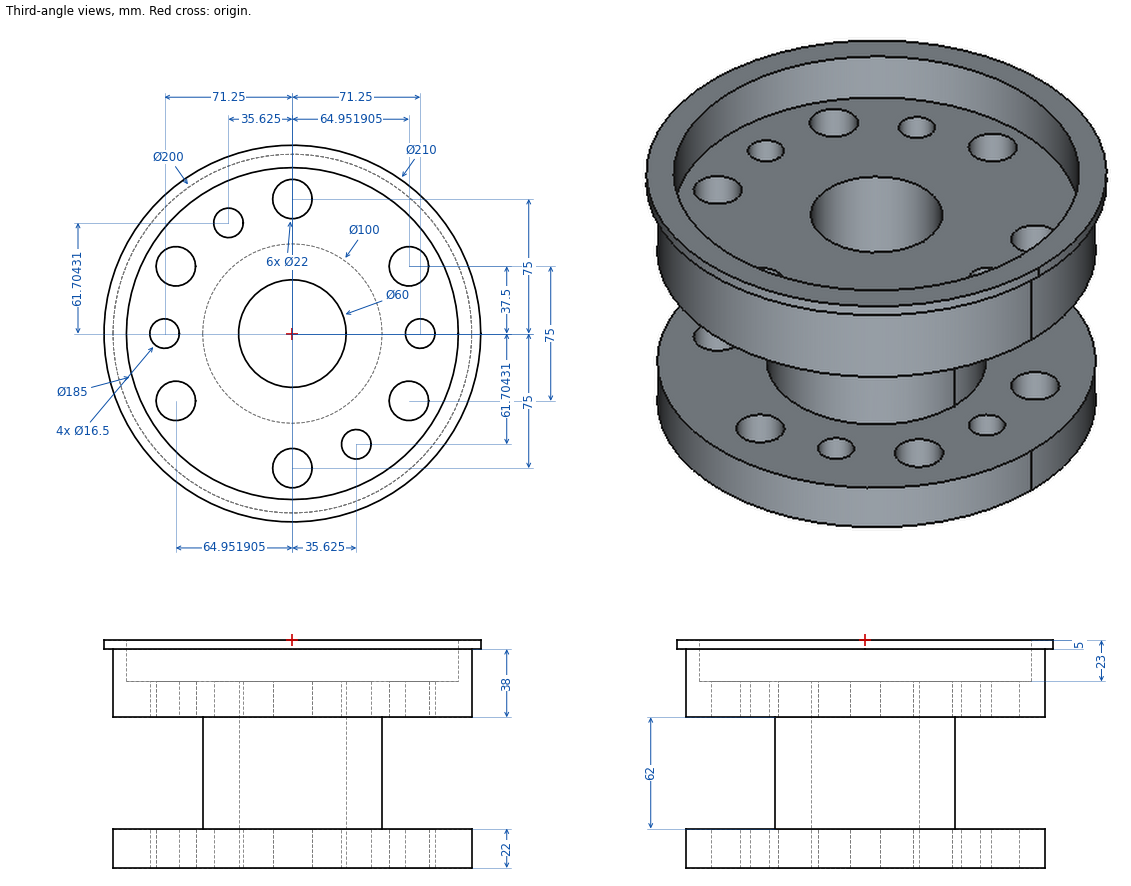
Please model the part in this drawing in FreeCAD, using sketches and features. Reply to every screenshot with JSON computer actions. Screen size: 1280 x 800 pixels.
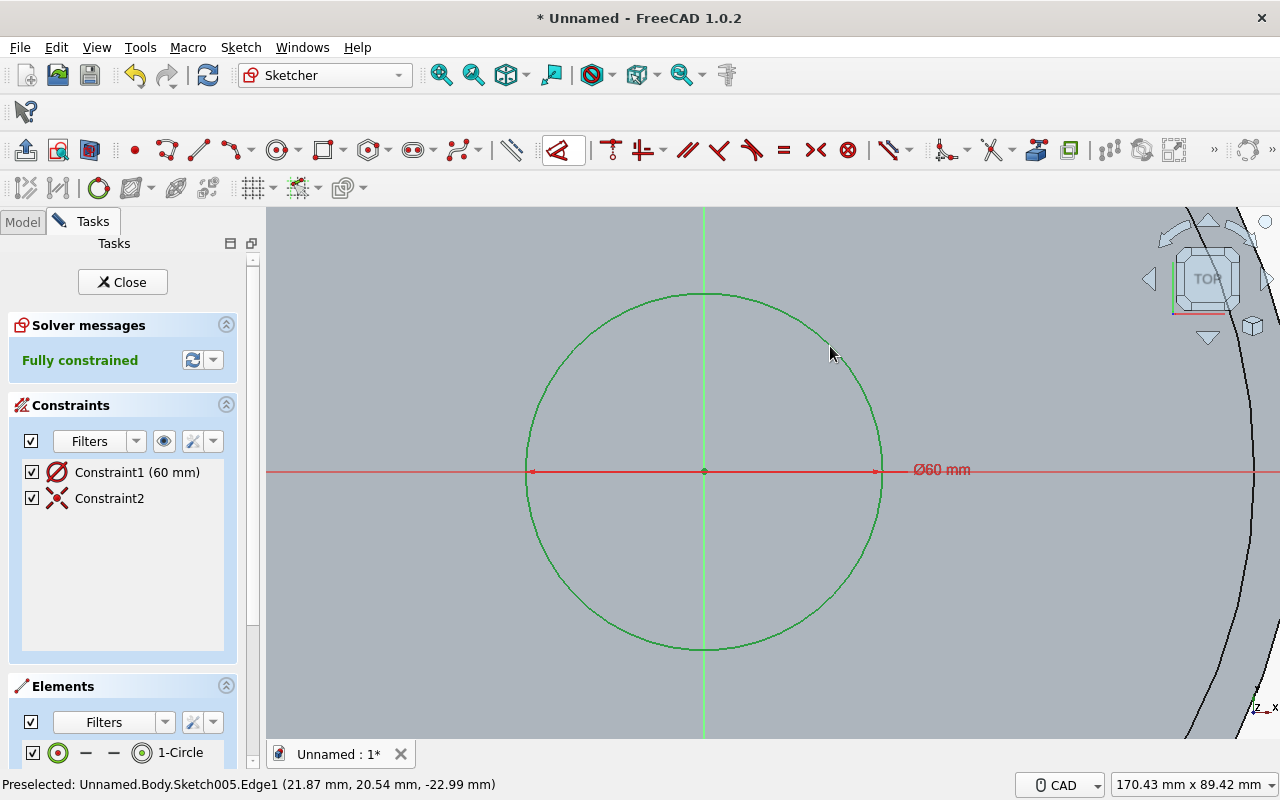
{"action": "left_click", "coordinate": [123, 282]}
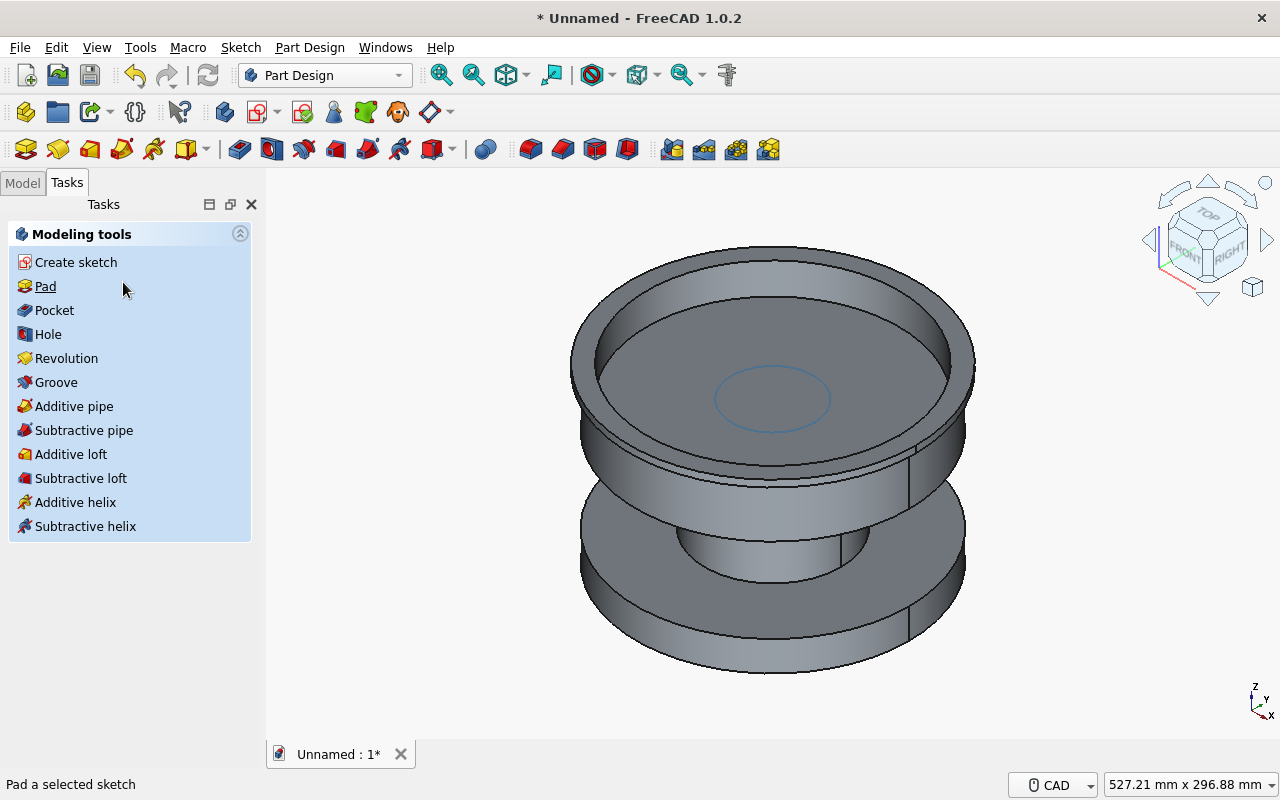
{"action": "left_click", "coordinate": [240, 150]}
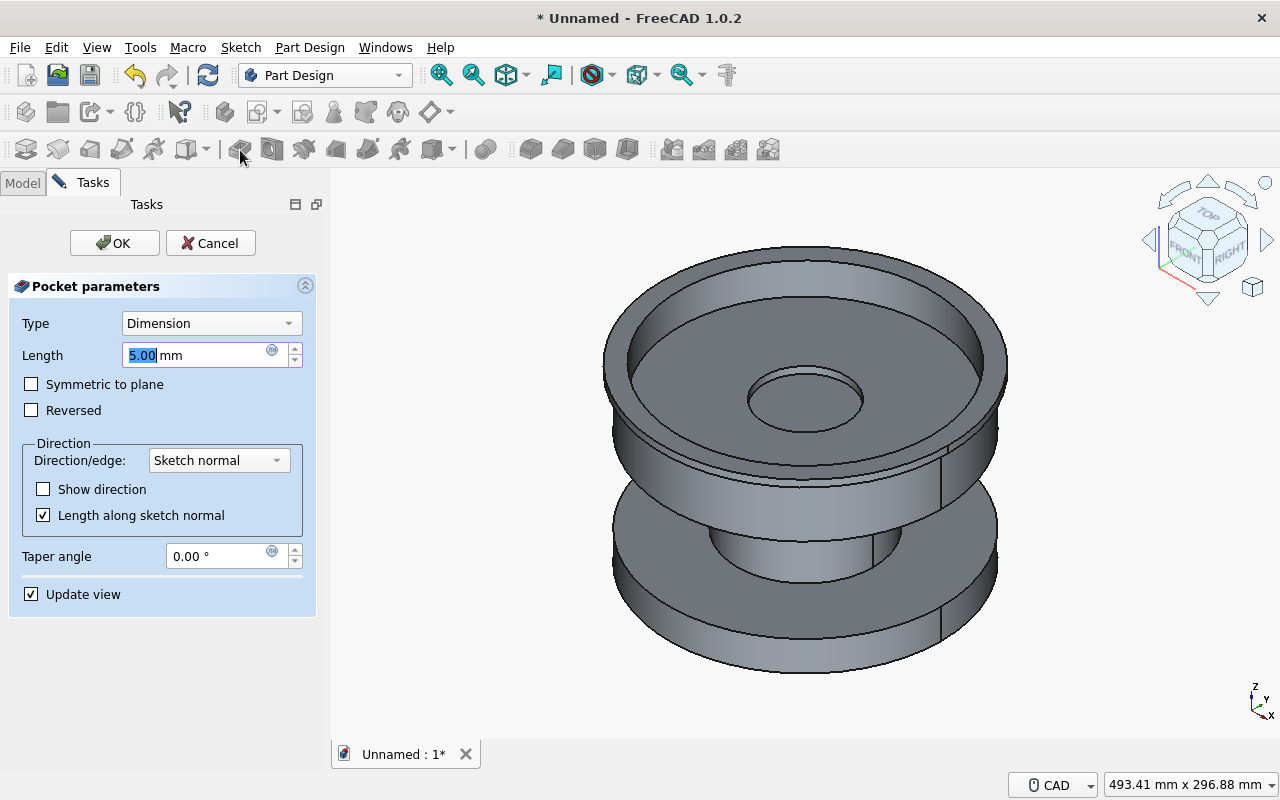
{"action": "left_click", "coordinate": [212, 324]}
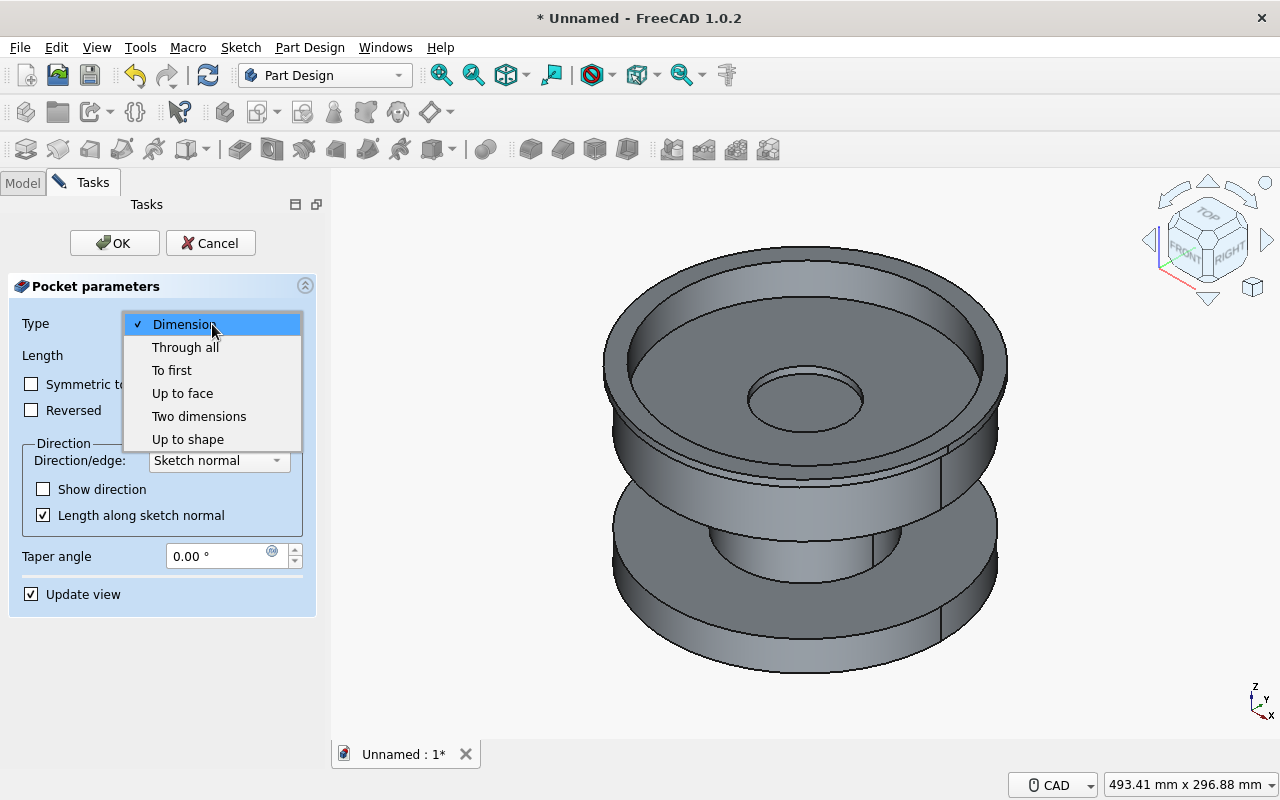
{"action": "left_click", "coordinate": [212, 348]}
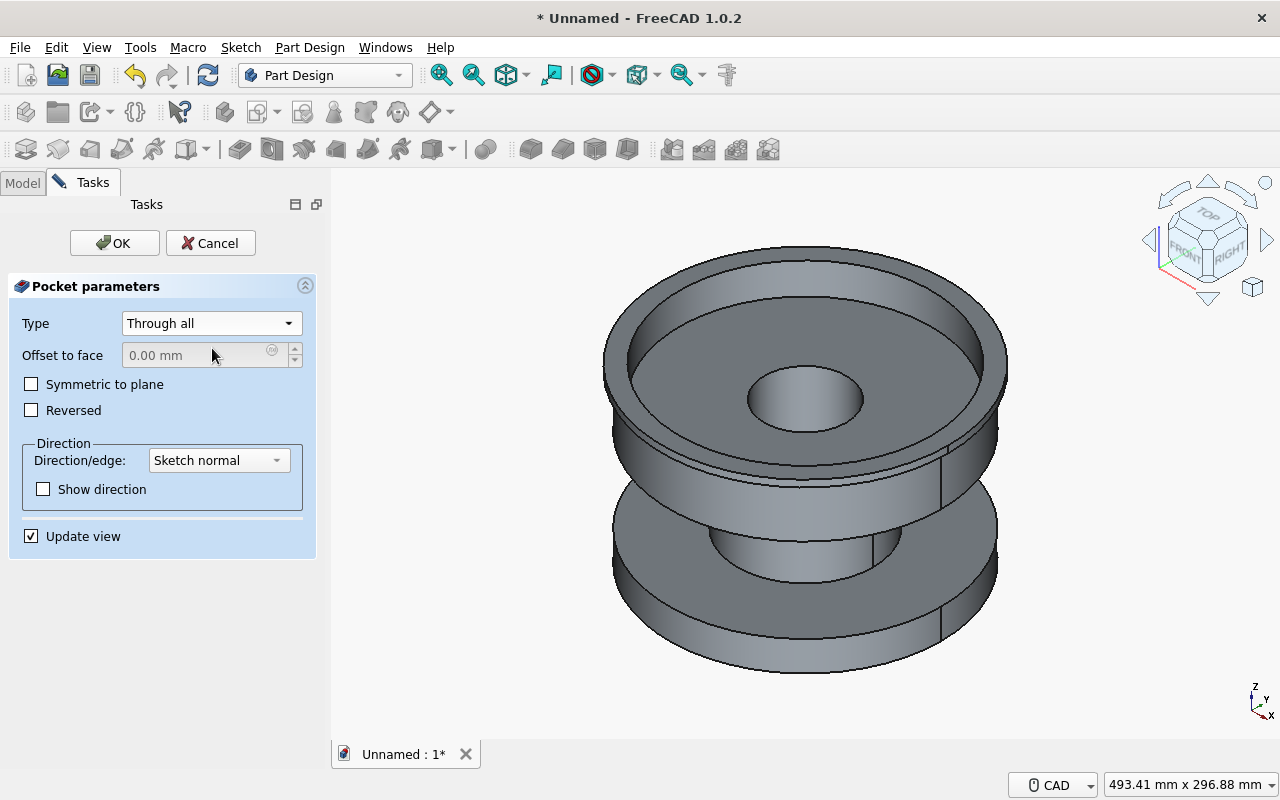
{"action": "left_click", "coordinate": [115, 243]}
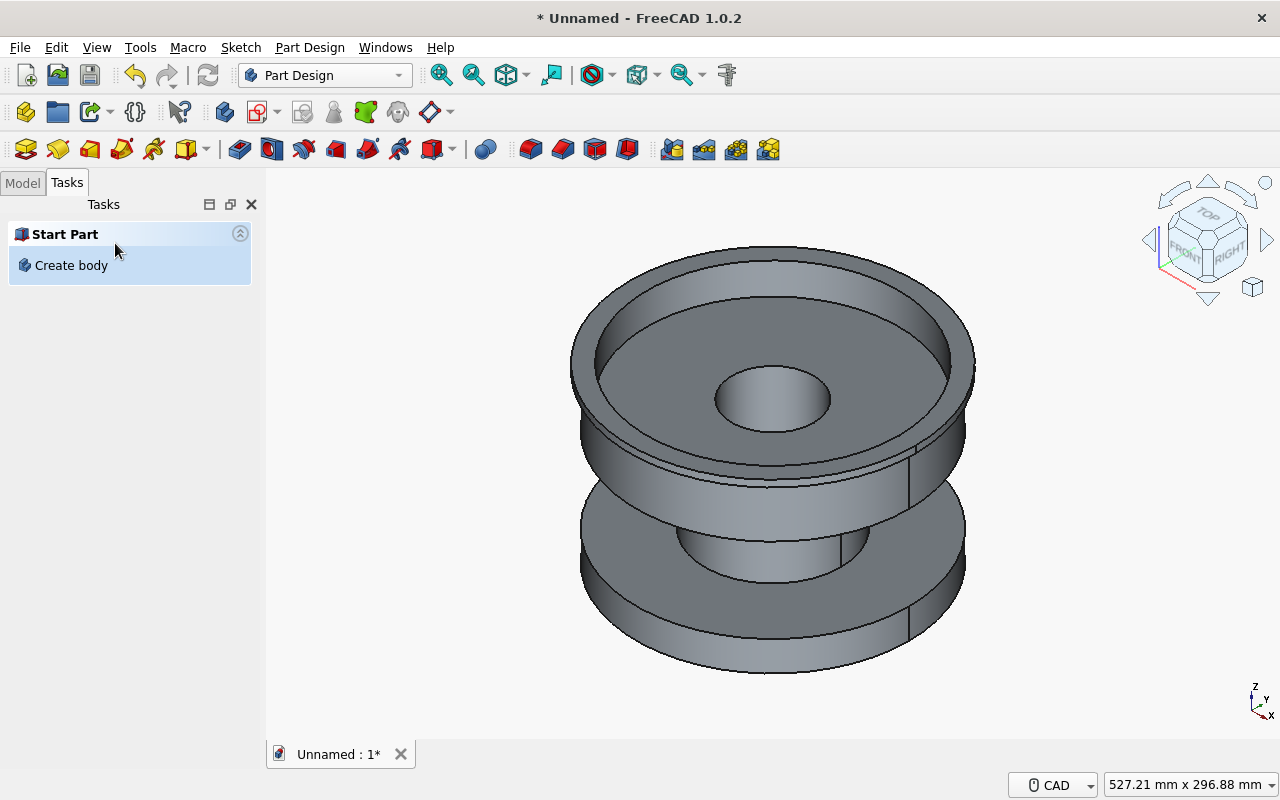
{"action": "left_click", "coordinate": [665, 419]}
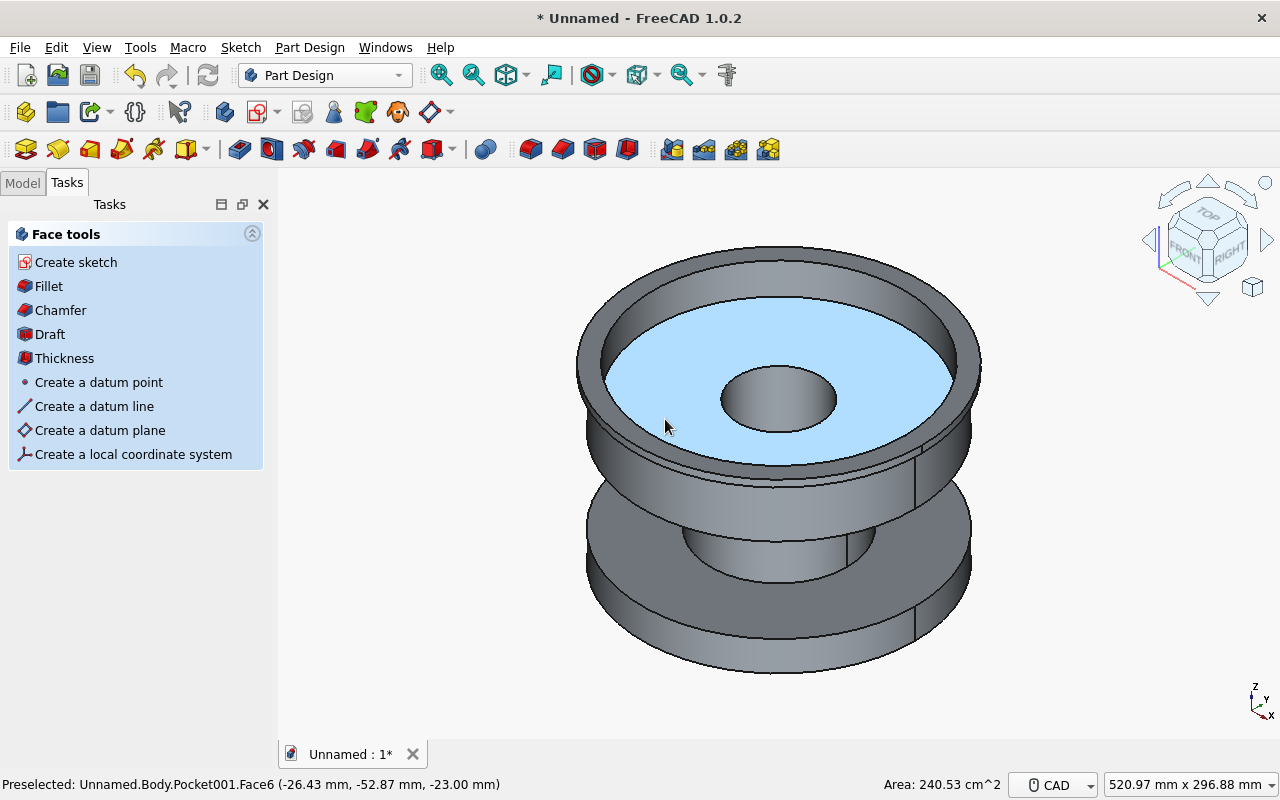
{"action": "left_click", "coordinate": [258, 112]}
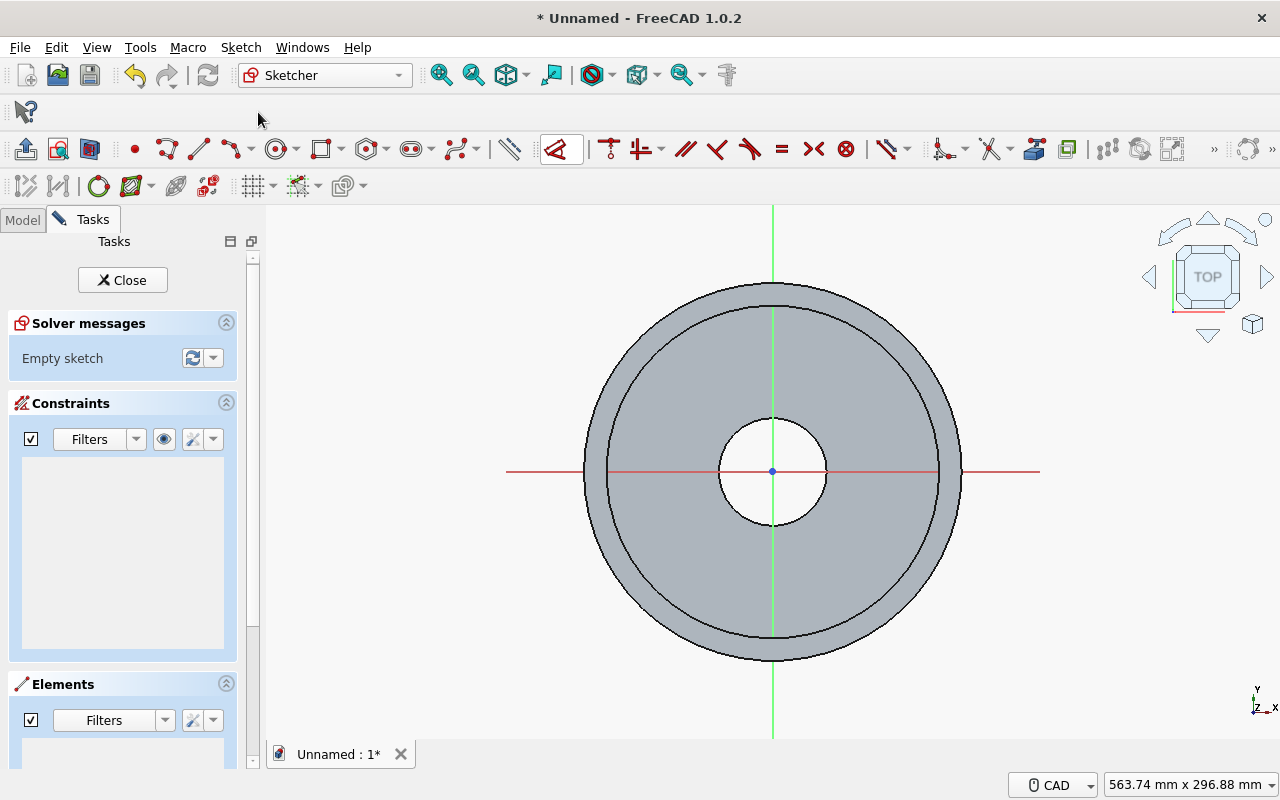
{"action": "left_click", "coordinate": [276, 150]}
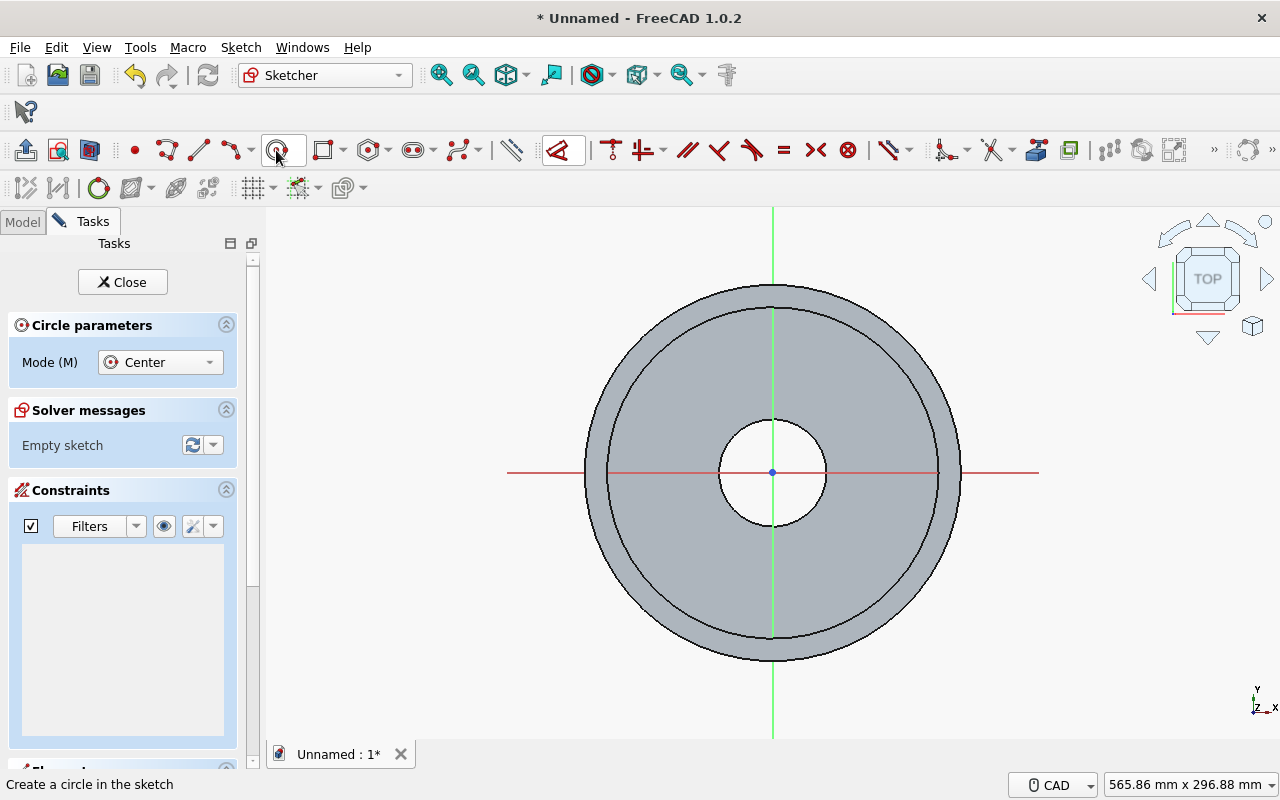
{"action": "left_click", "coordinate": [773, 339]}
{"action": "mouse_move", "coordinate": [791, 332]}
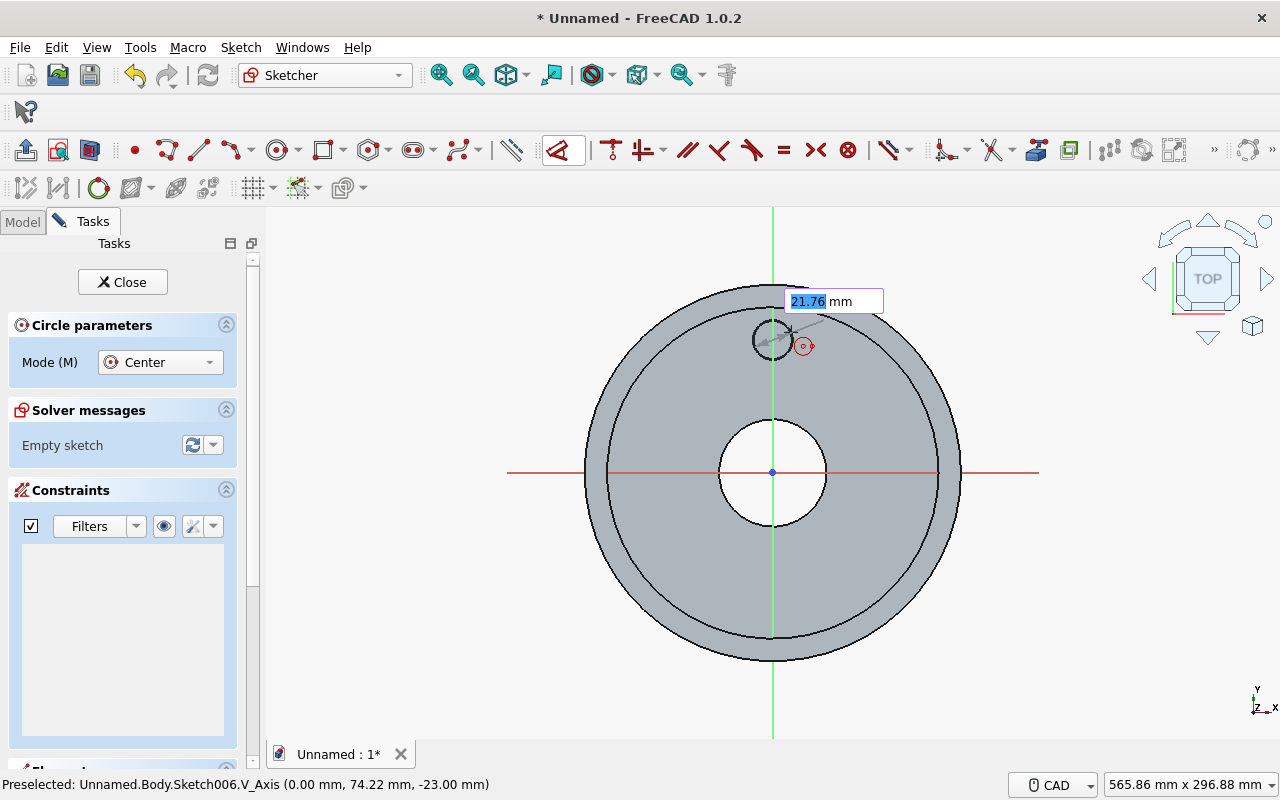
{"action": "type", "text": "22"}
{"action": "key", "text": "Return"}